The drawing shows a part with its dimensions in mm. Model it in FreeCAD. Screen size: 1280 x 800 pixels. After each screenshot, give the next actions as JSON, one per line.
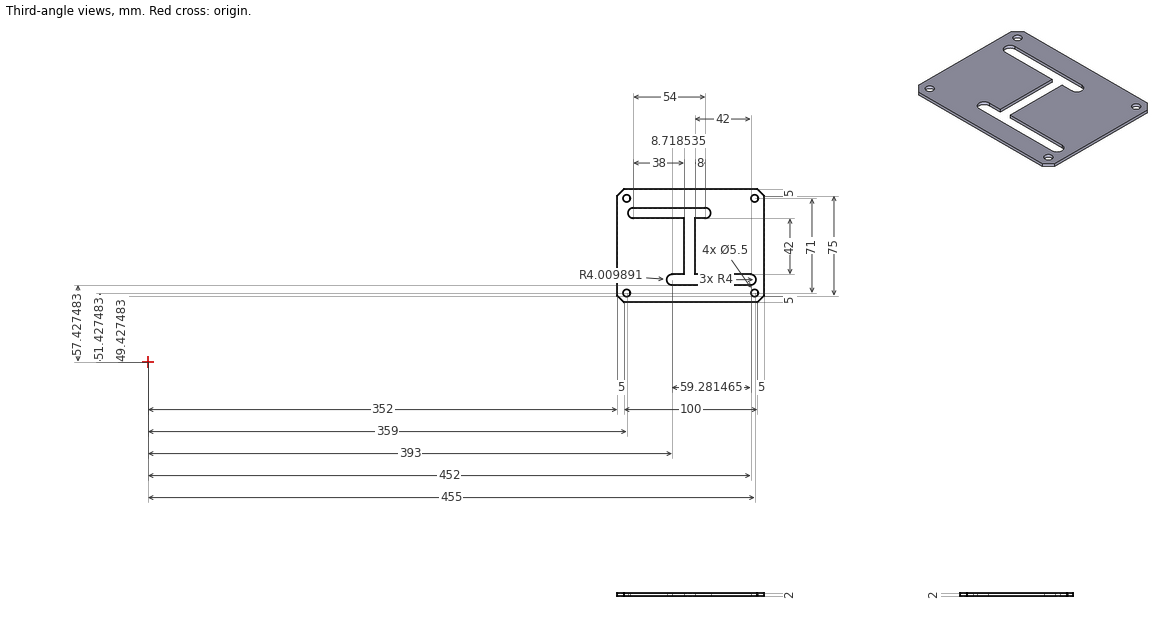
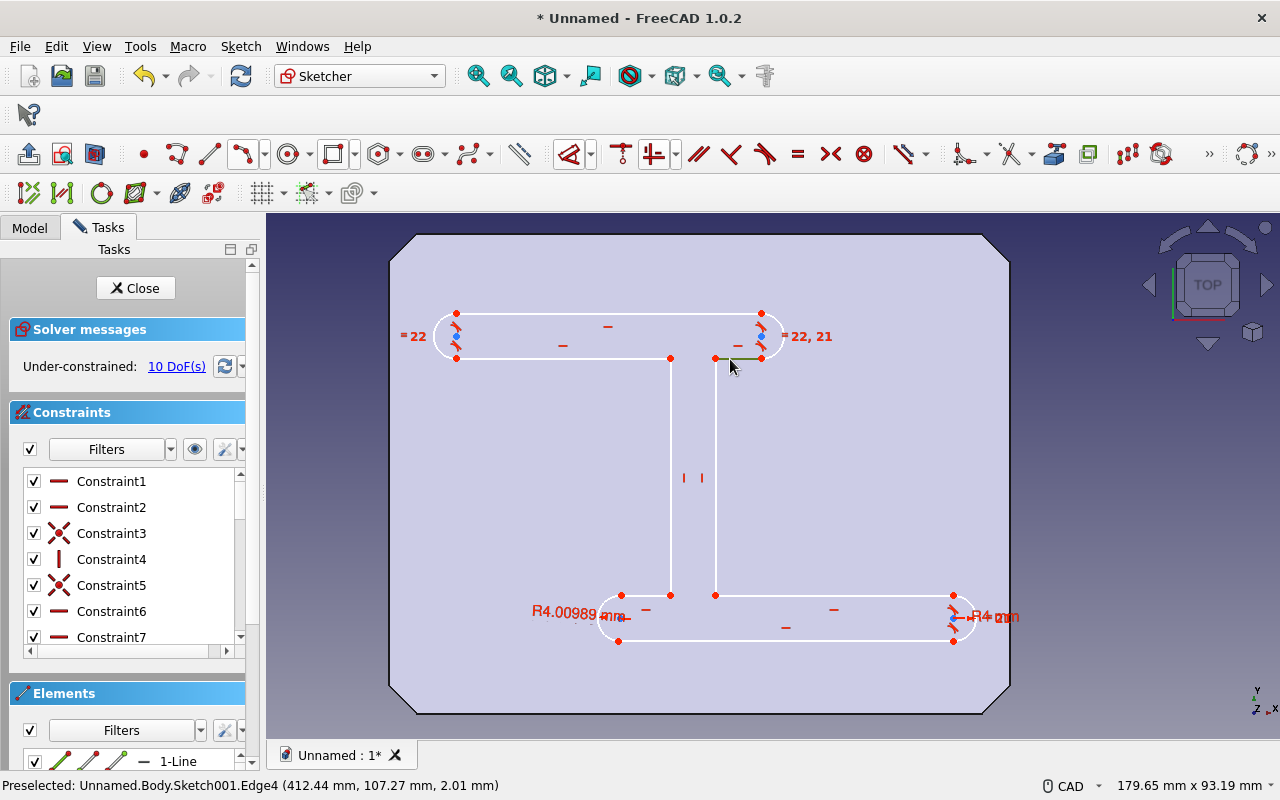
{"action": "key", "text": "l"}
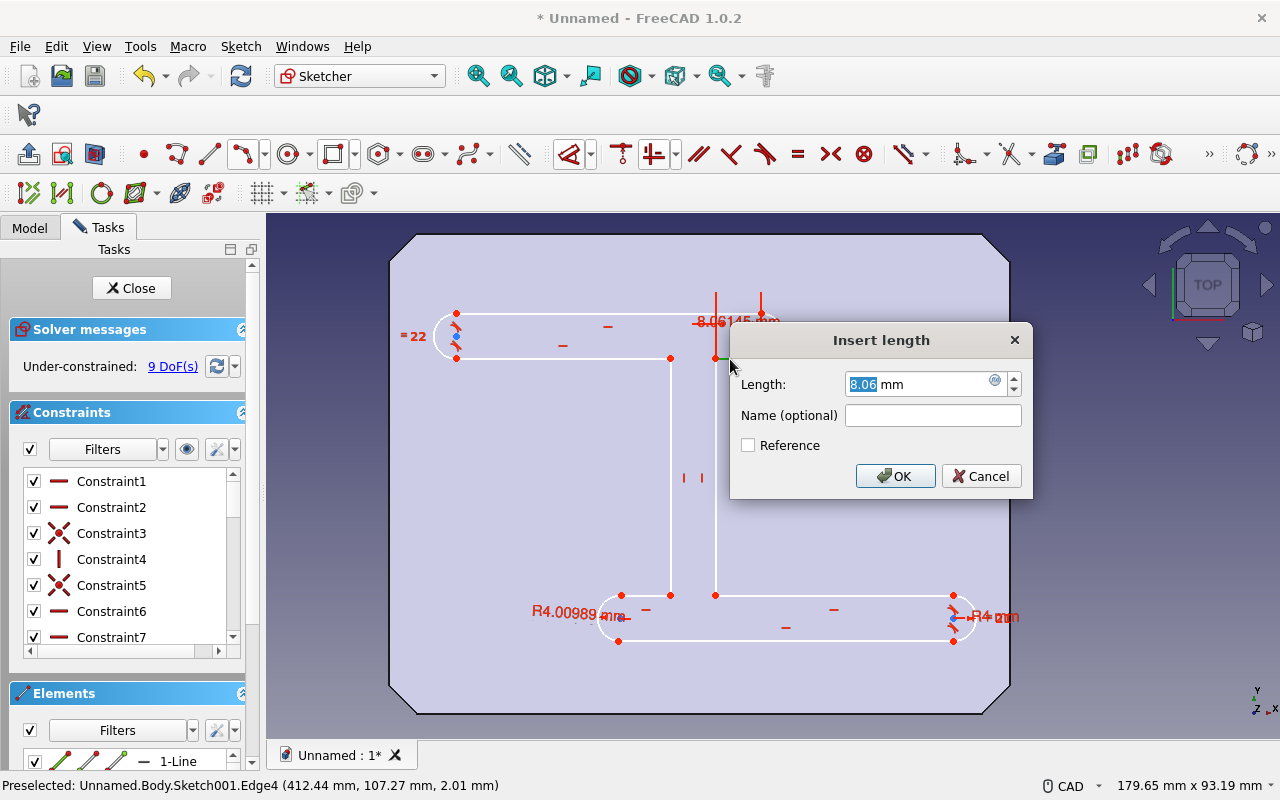
{"action": "type", "text": "8"}
{"action": "key", "text": "Return"}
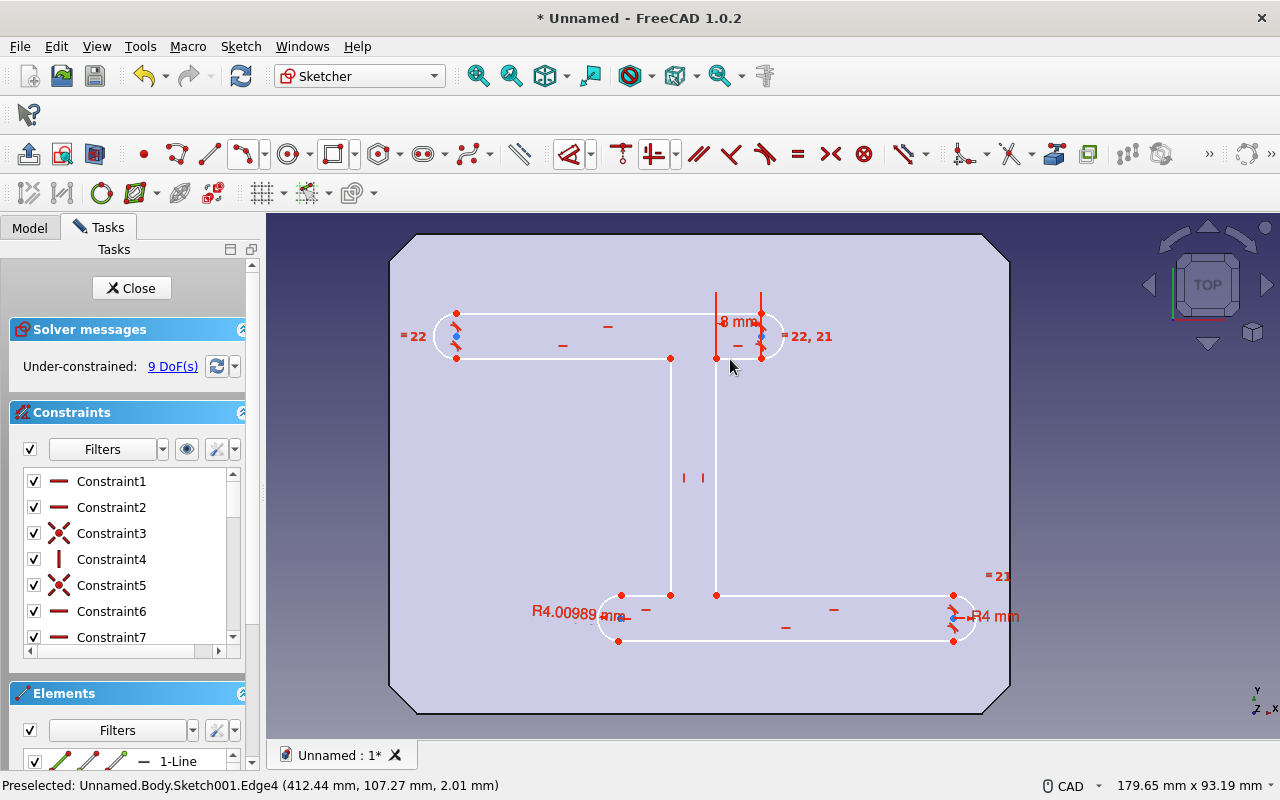
{"action": "left_click", "coordinate": [882, 596]}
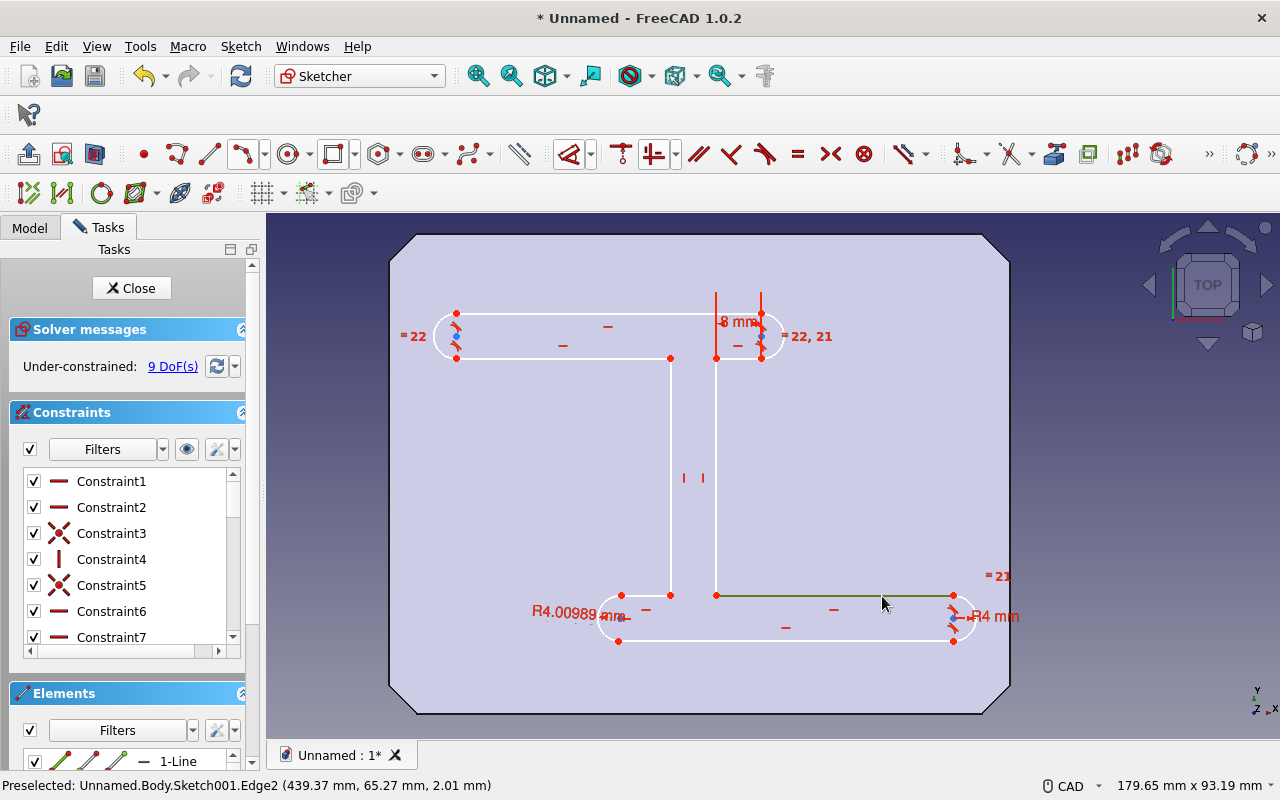
{"action": "left_click", "coordinate": [590, 154]}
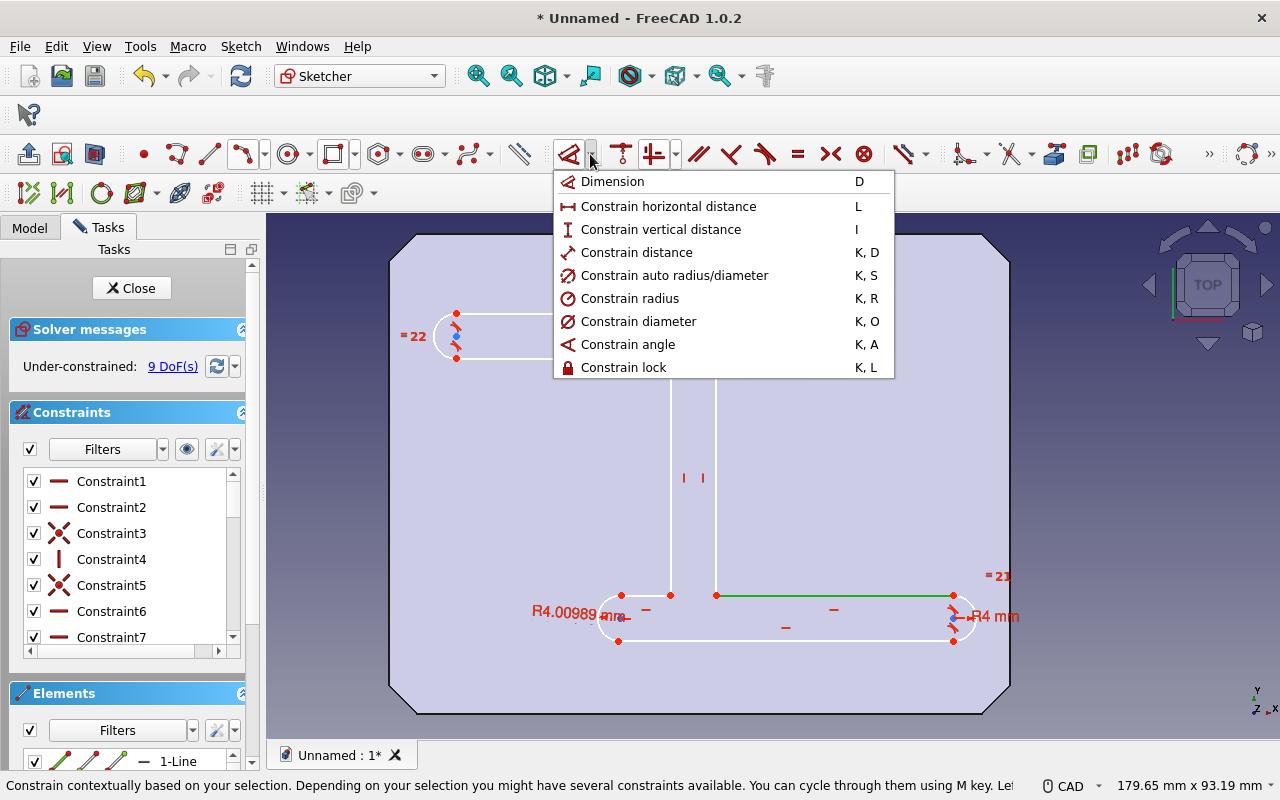
{"action": "left_click", "coordinate": [724, 206]}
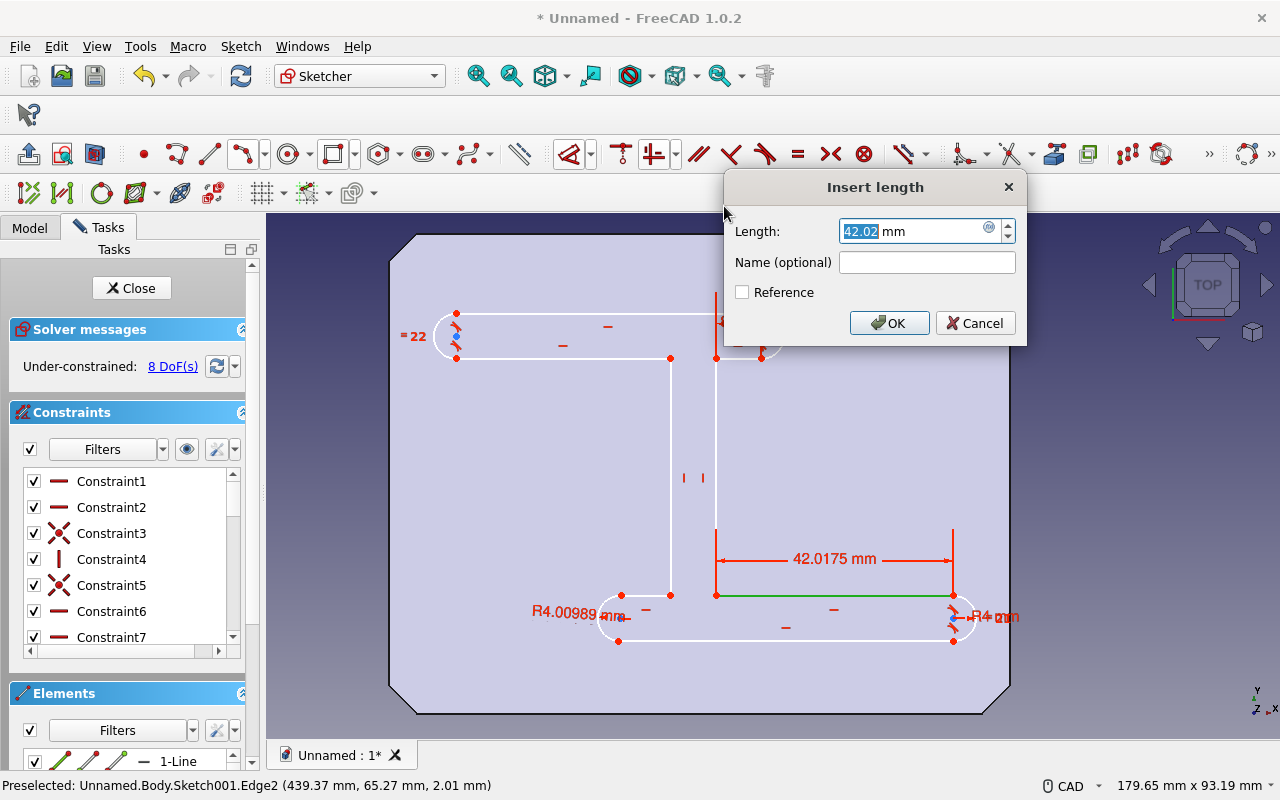
{"action": "type", "text": "42"}
{"action": "key", "text": "Return"}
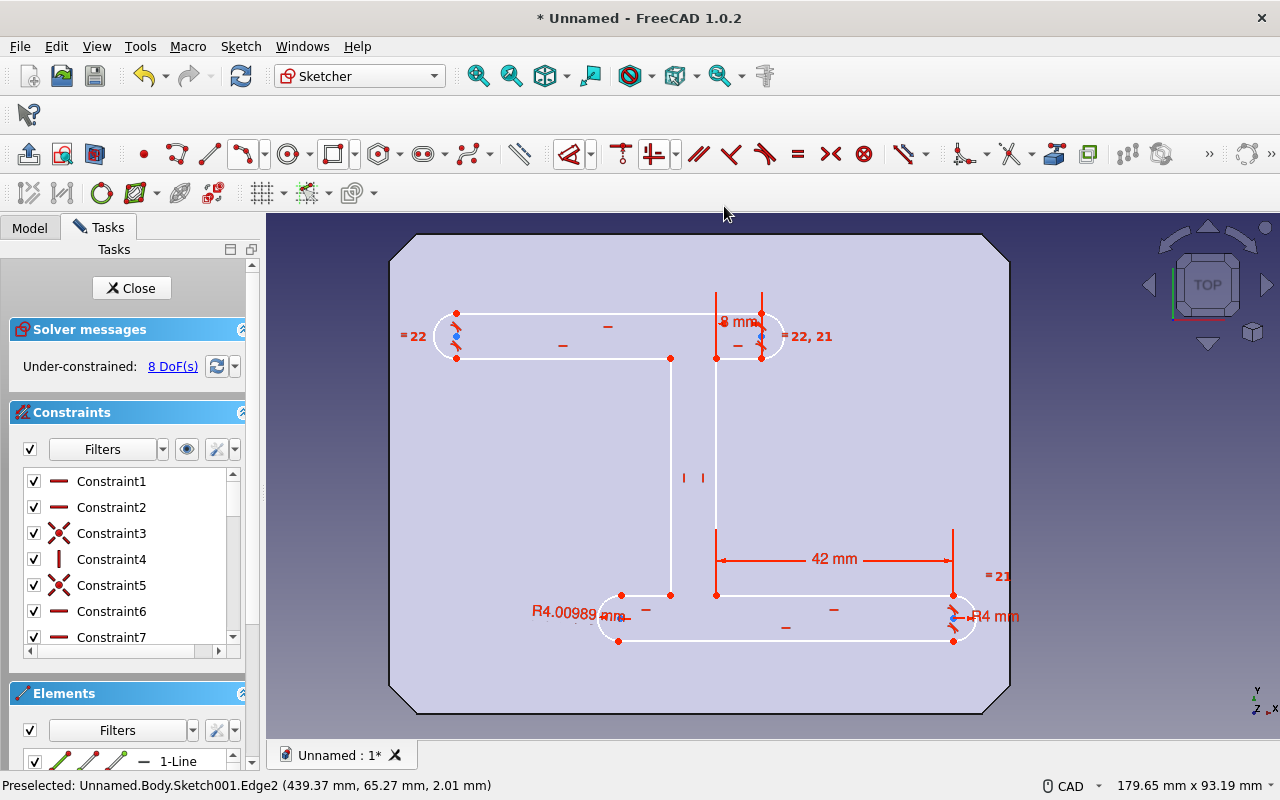
{"action": "left_click", "coordinate": [716, 525]}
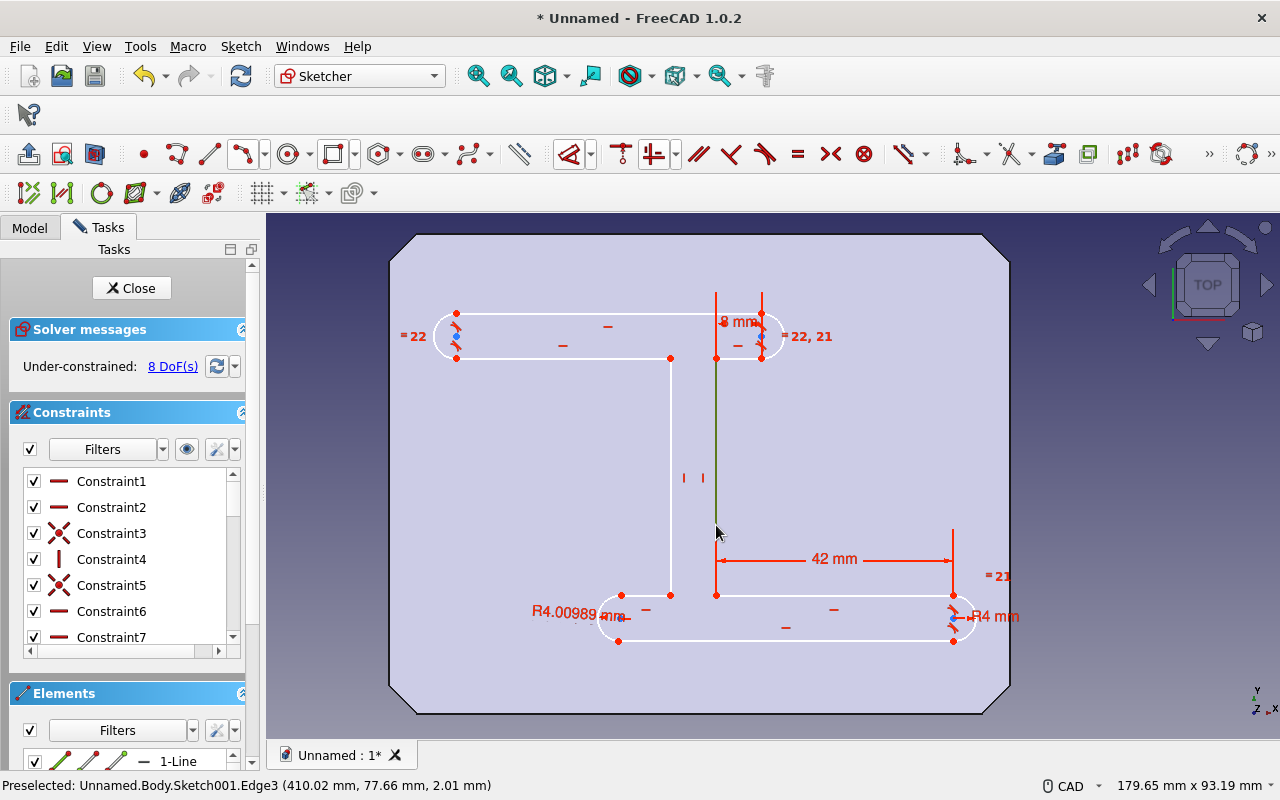
{"action": "left_click", "coordinate": [590, 154]}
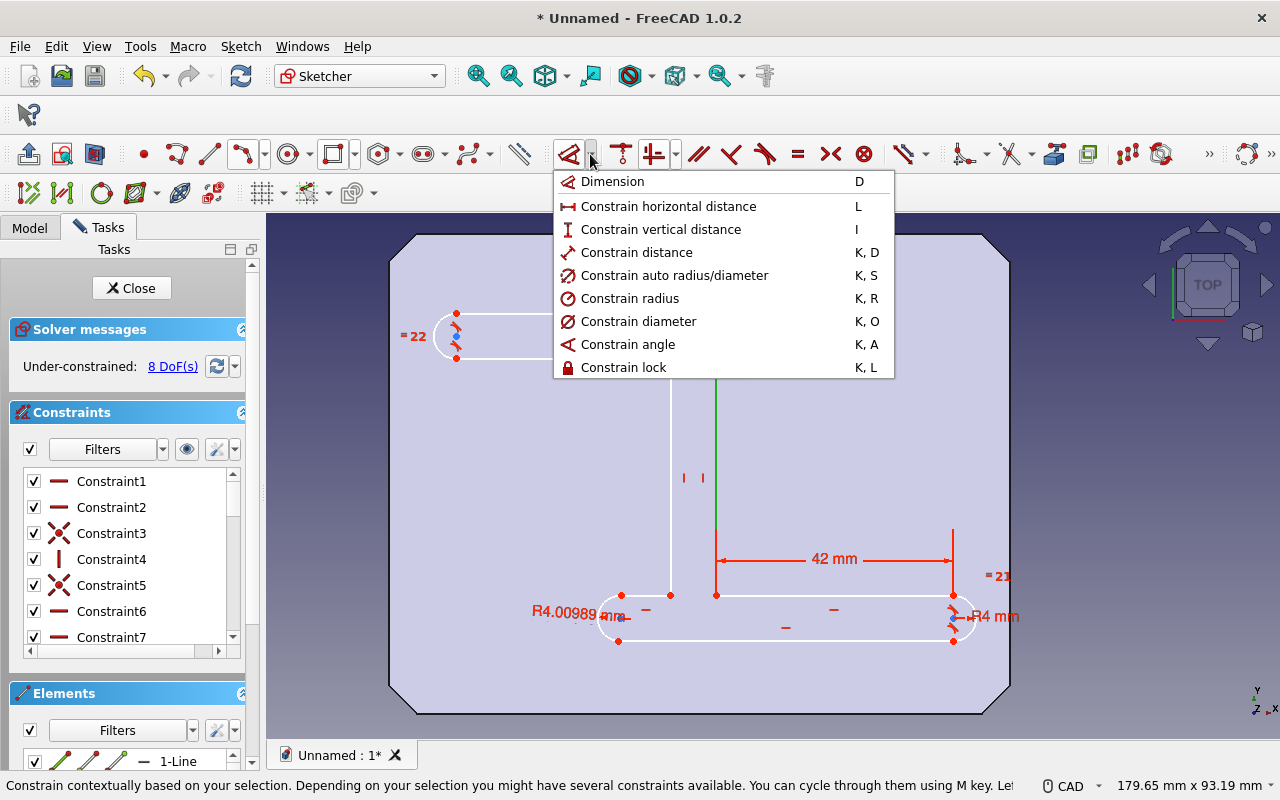
{"action": "left_click", "coordinate": [724, 230]}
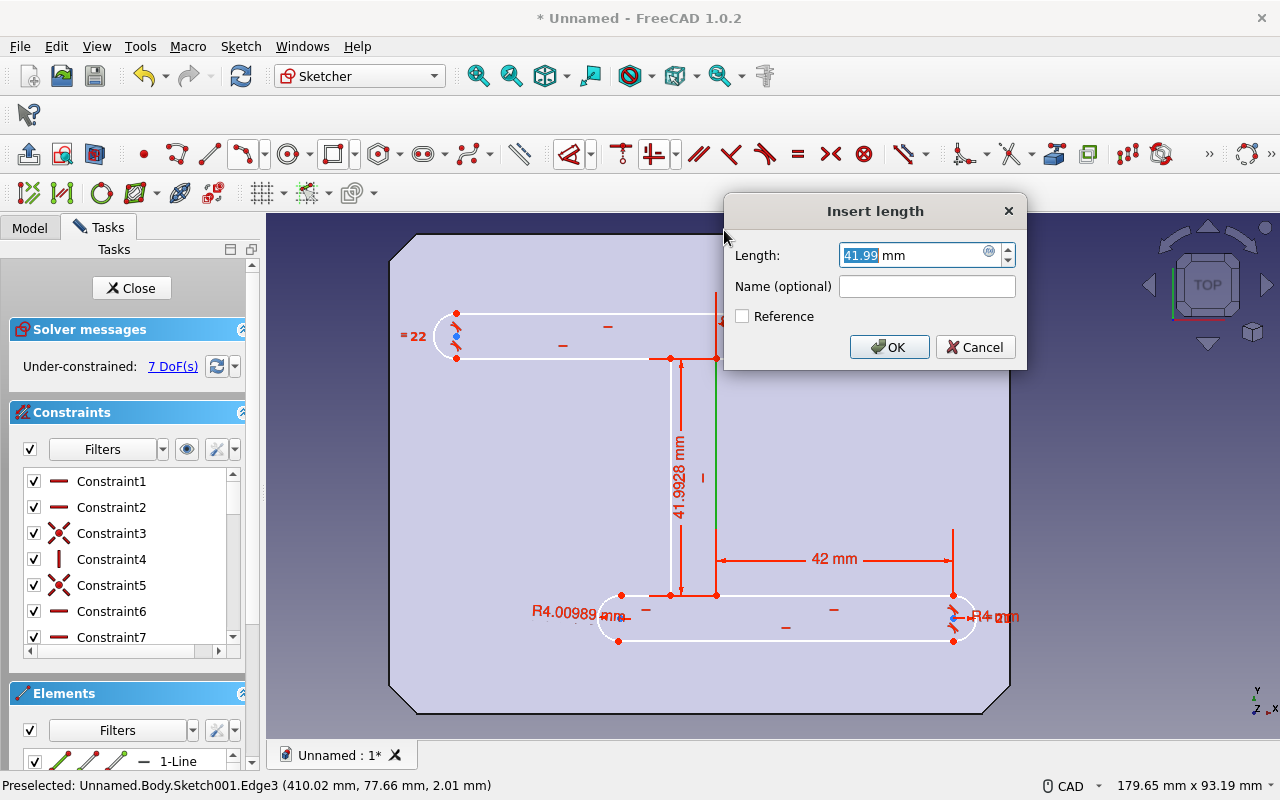
{"action": "type", "text": "42"}
{"action": "key", "text": "Return"}